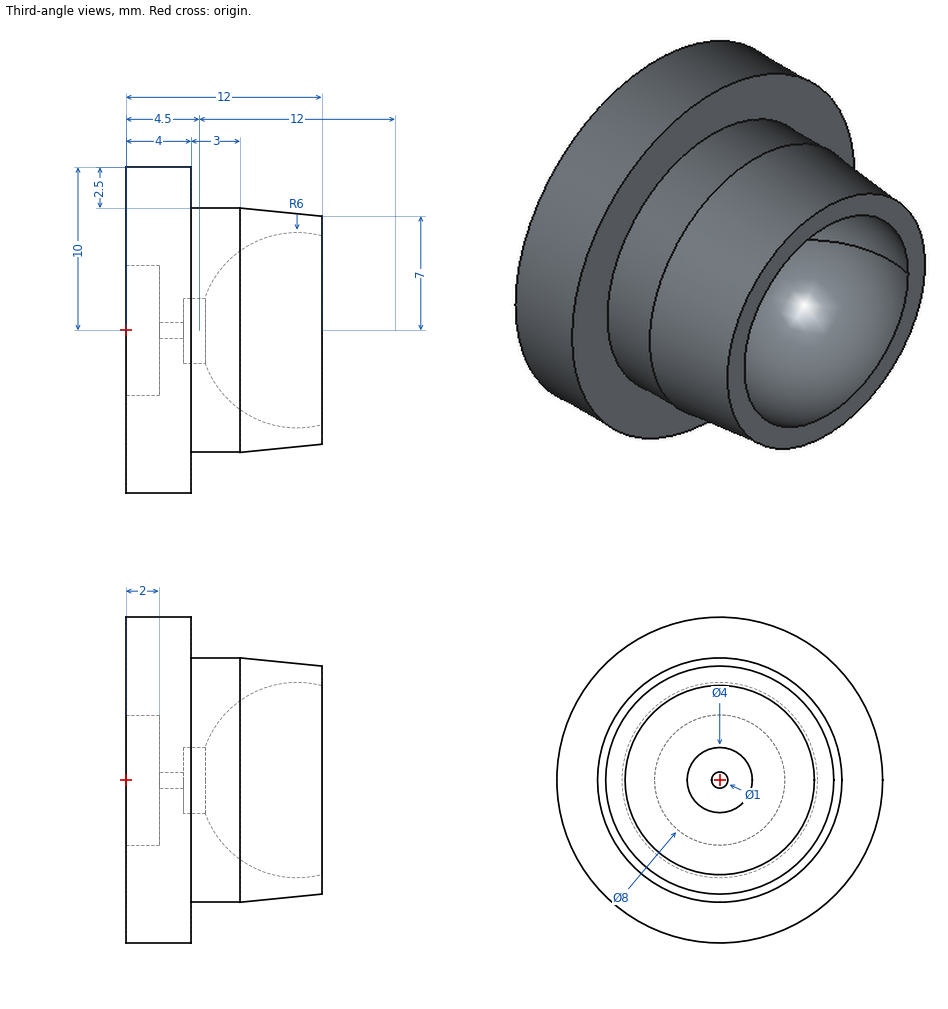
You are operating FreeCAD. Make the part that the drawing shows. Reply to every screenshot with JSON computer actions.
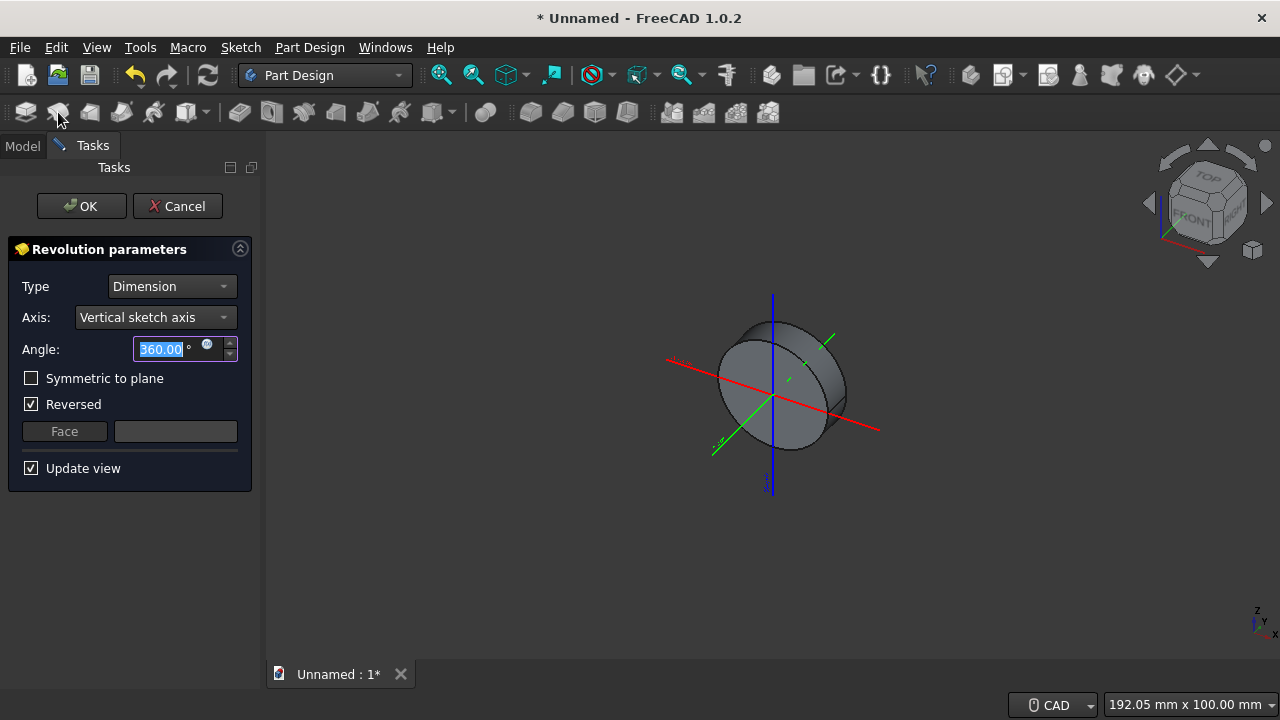
{"action": "left_click", "coordinate": [156, 318]}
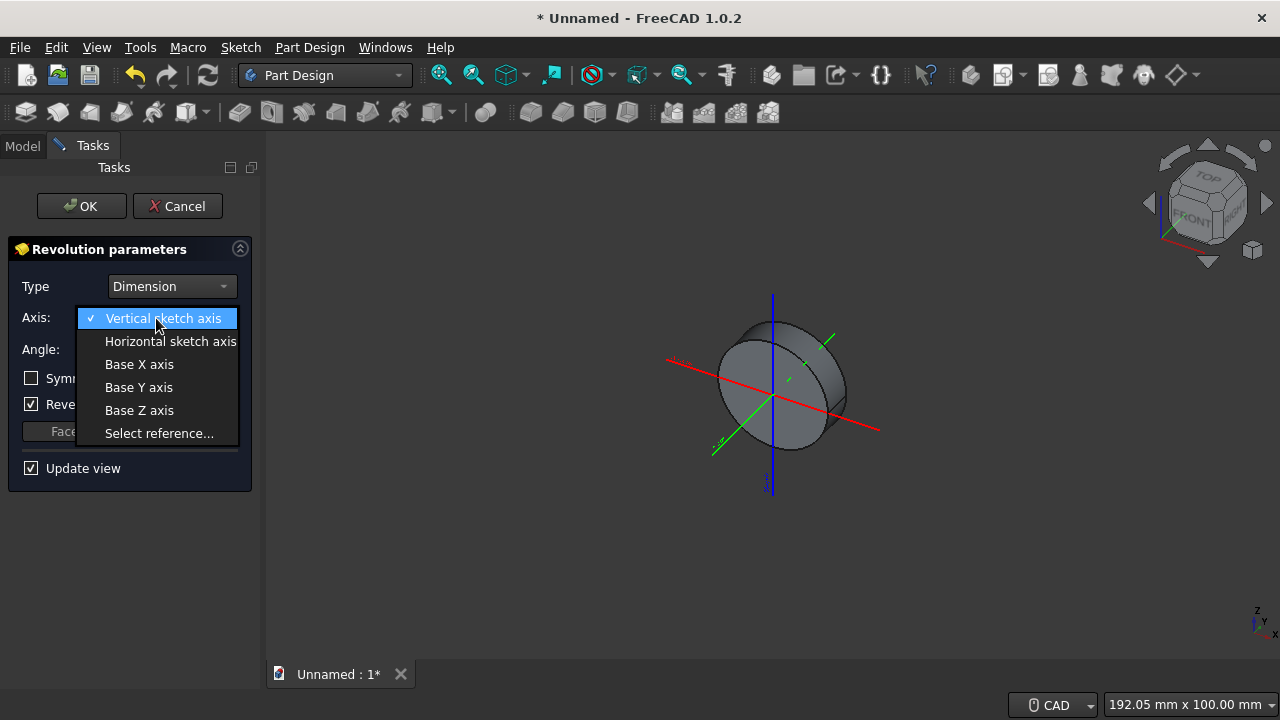
{"action": "left_click", "coordinate": [156, 342]}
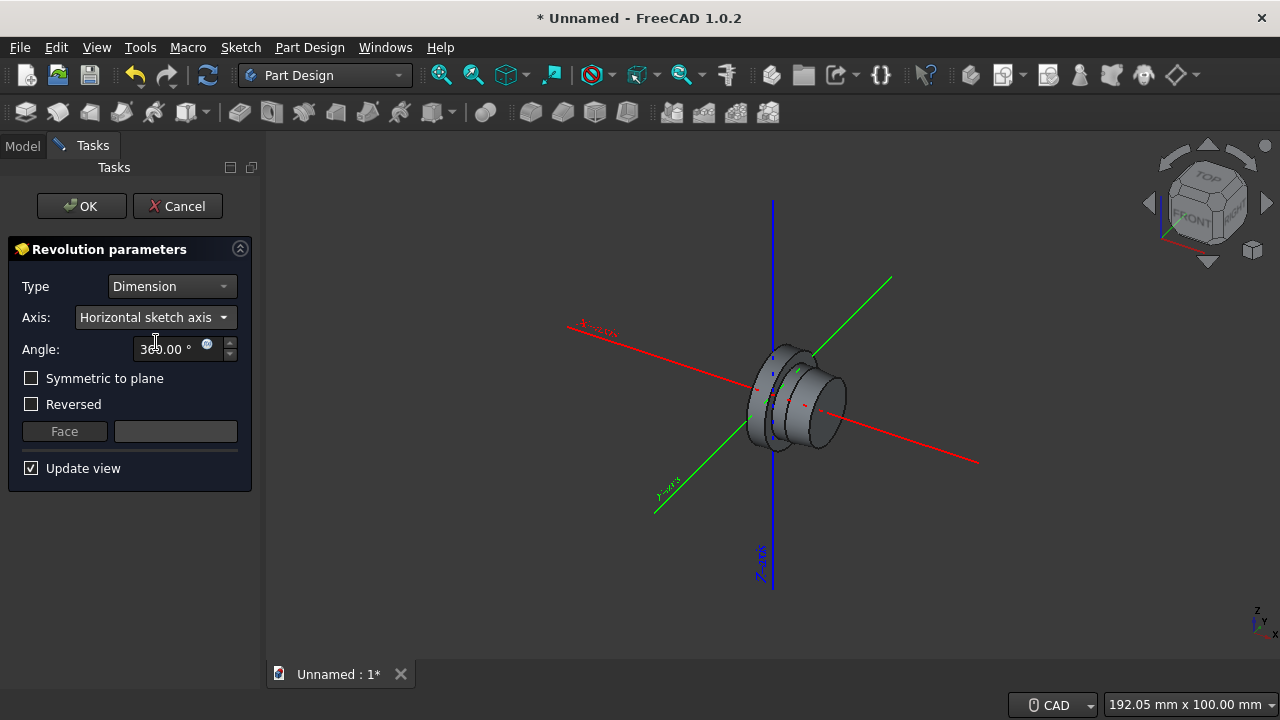
{"action": "left_click", "coordinate": [82, 206]}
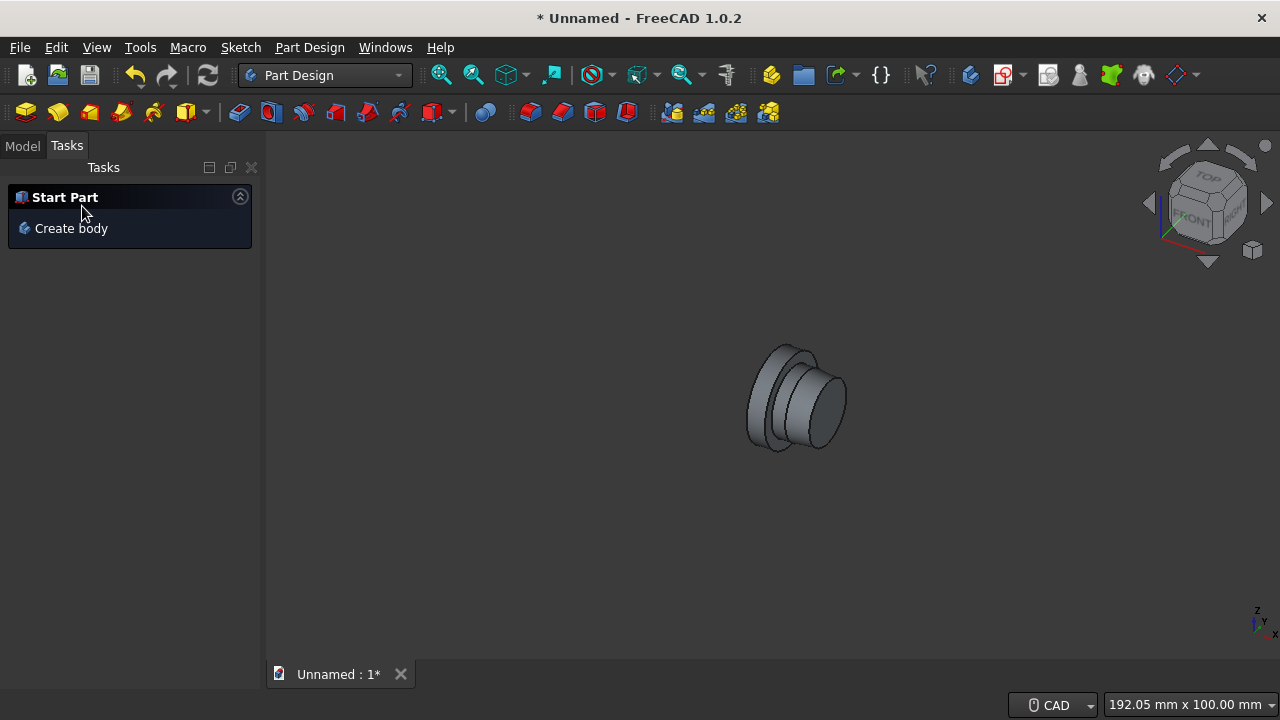
{"action": "left_click", "coordinate": [442, 76]}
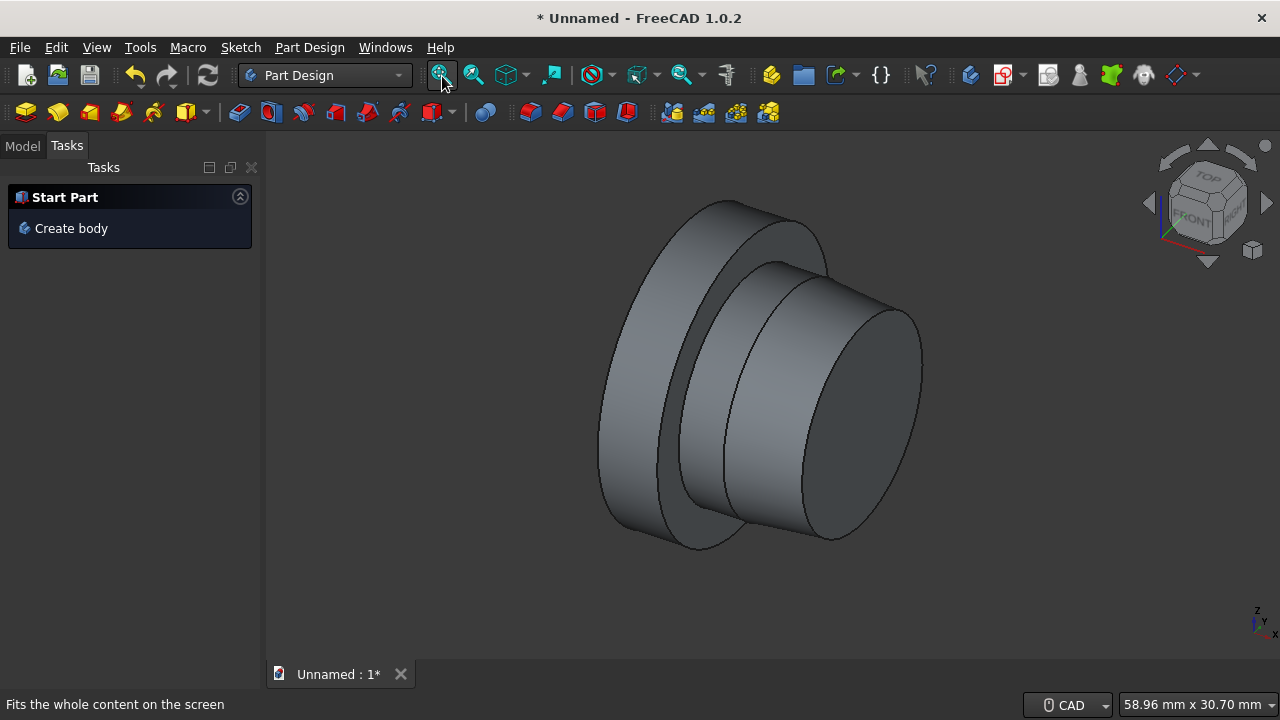
{"action": "key", "text": "6"}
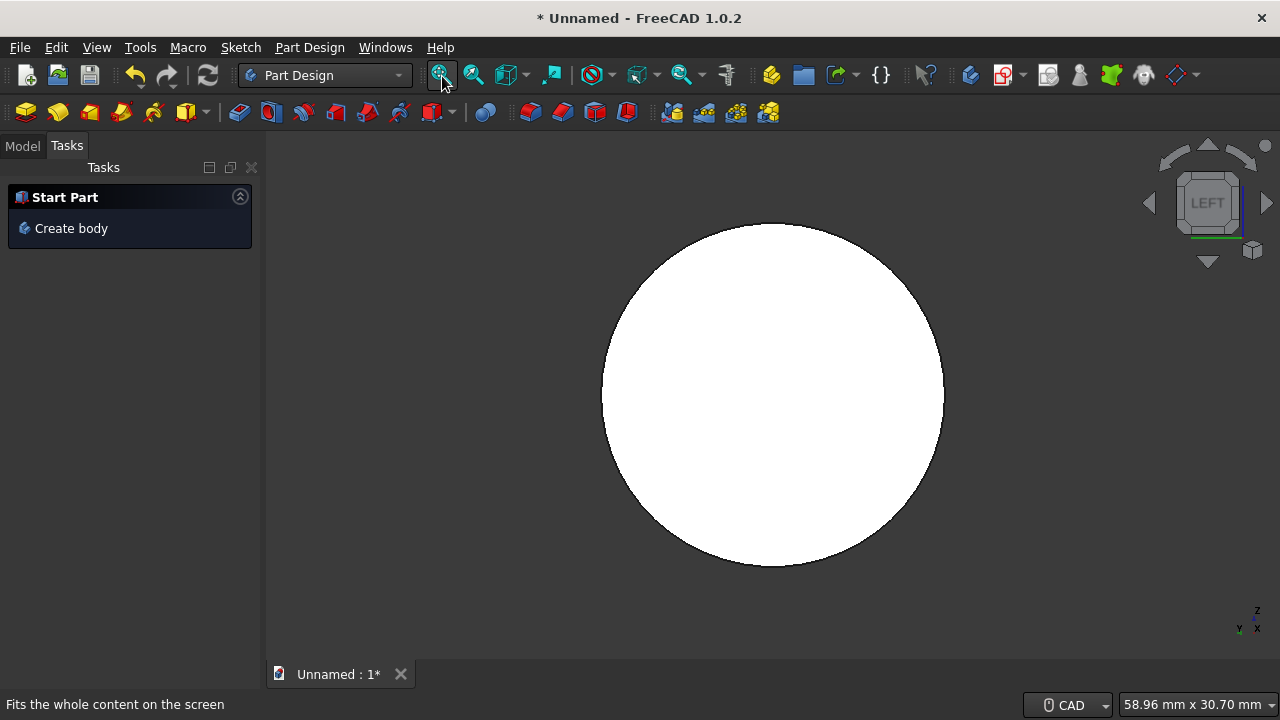
{"action": "left_click", "coordinate": [773, 394]}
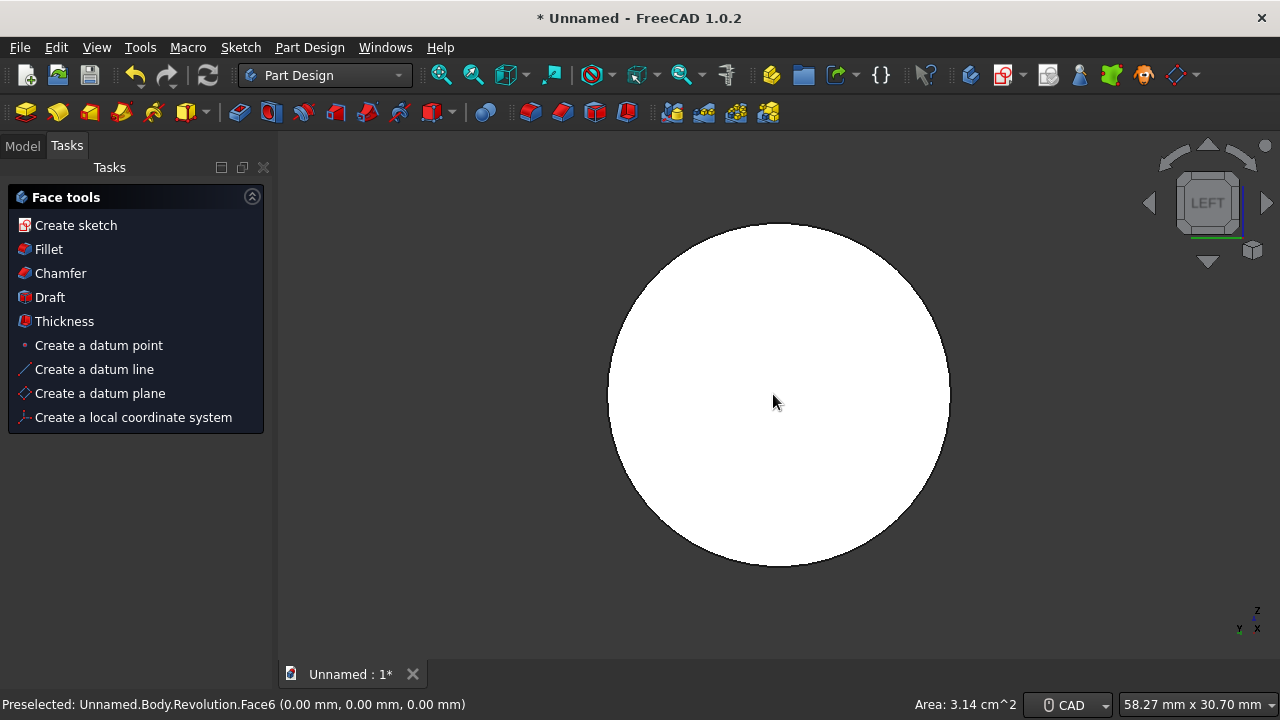
{"action": "left_click", "coordinate": [1004, 76]}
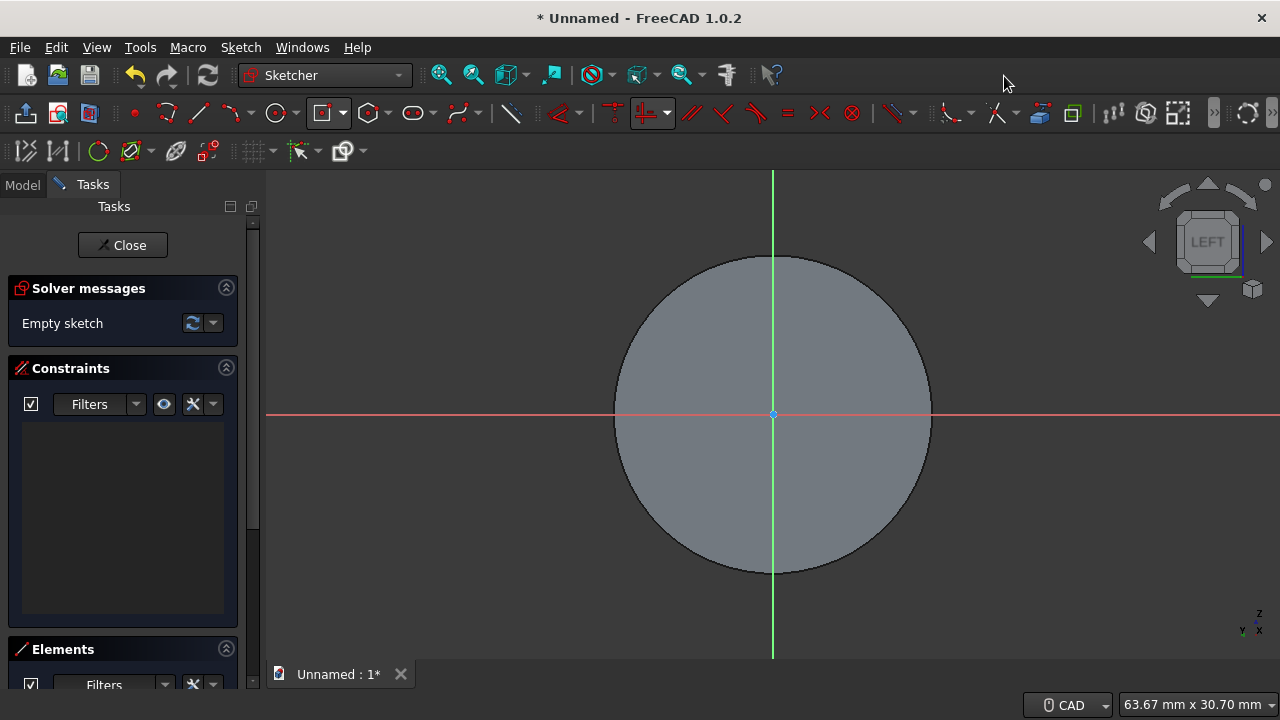
{"action": "scroll", "coordinate": [829, 414], "scroll_direction": "up", "scroll_amount": 4}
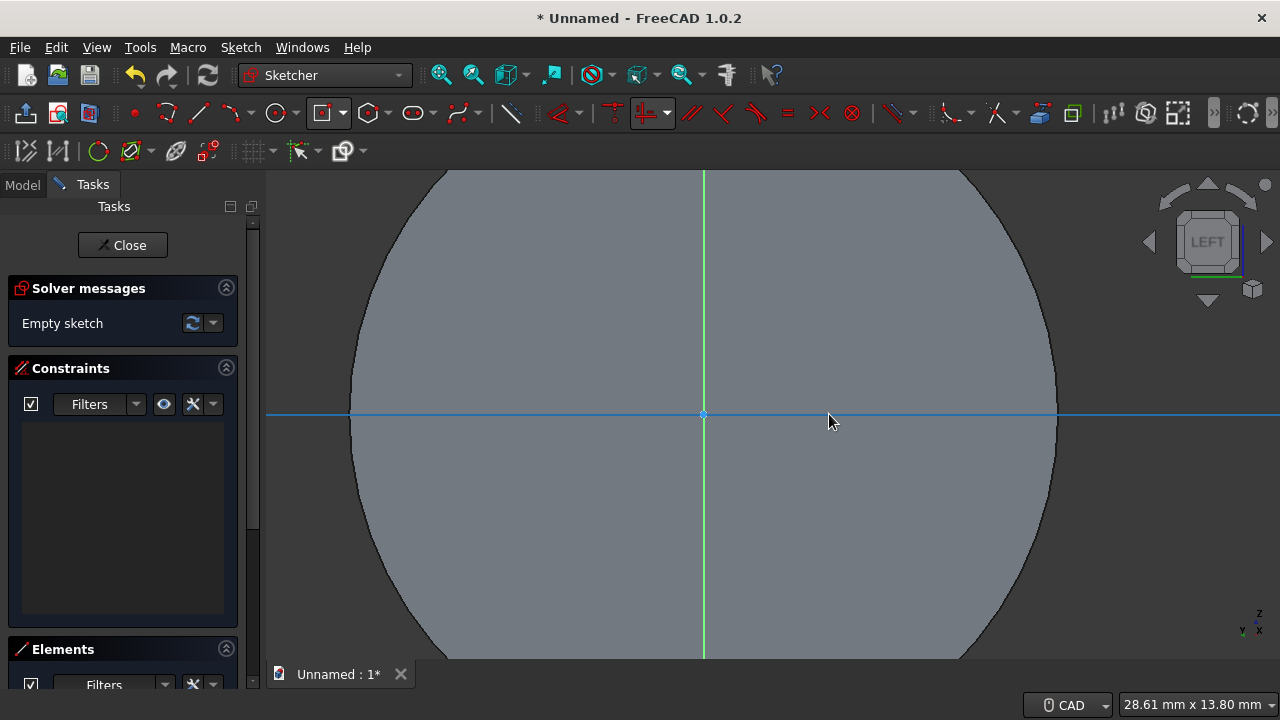
{"action": "left_click", "coordinate": [276, 114]}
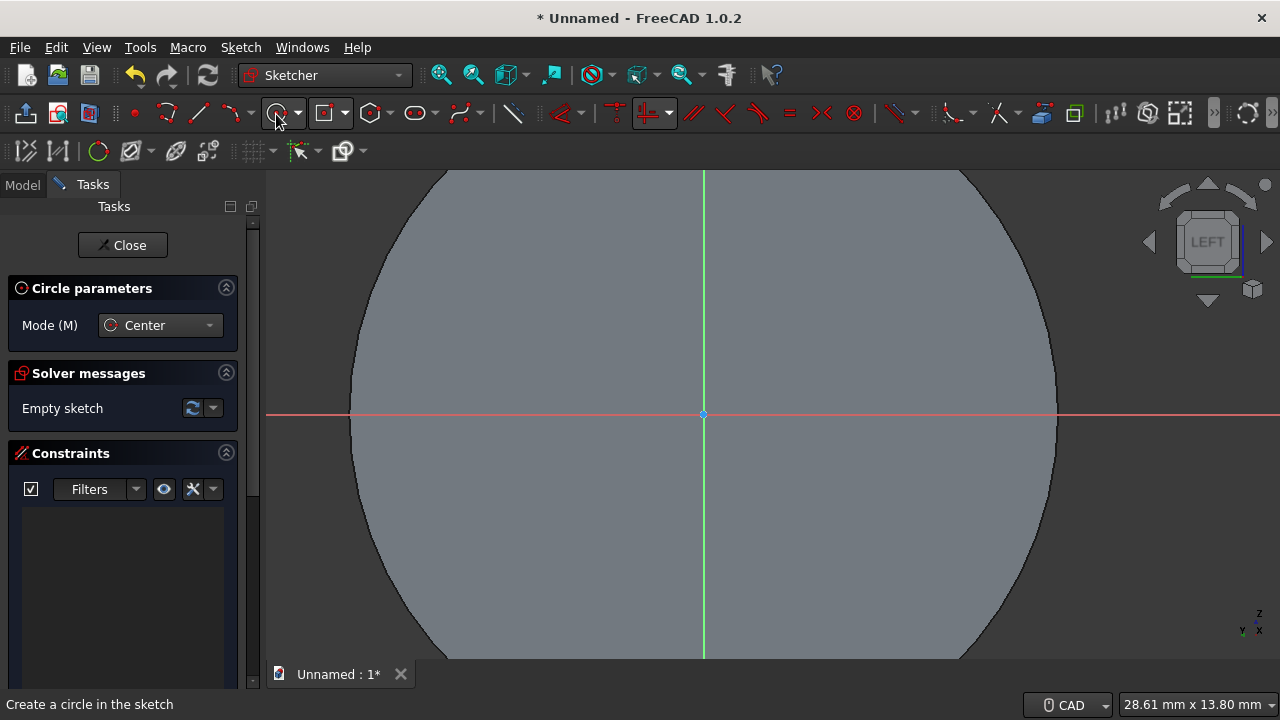
{"action": "left_click", "coordinate": [704, 414]}
{"action": "mouse_move", "coordinate": [804, 314]}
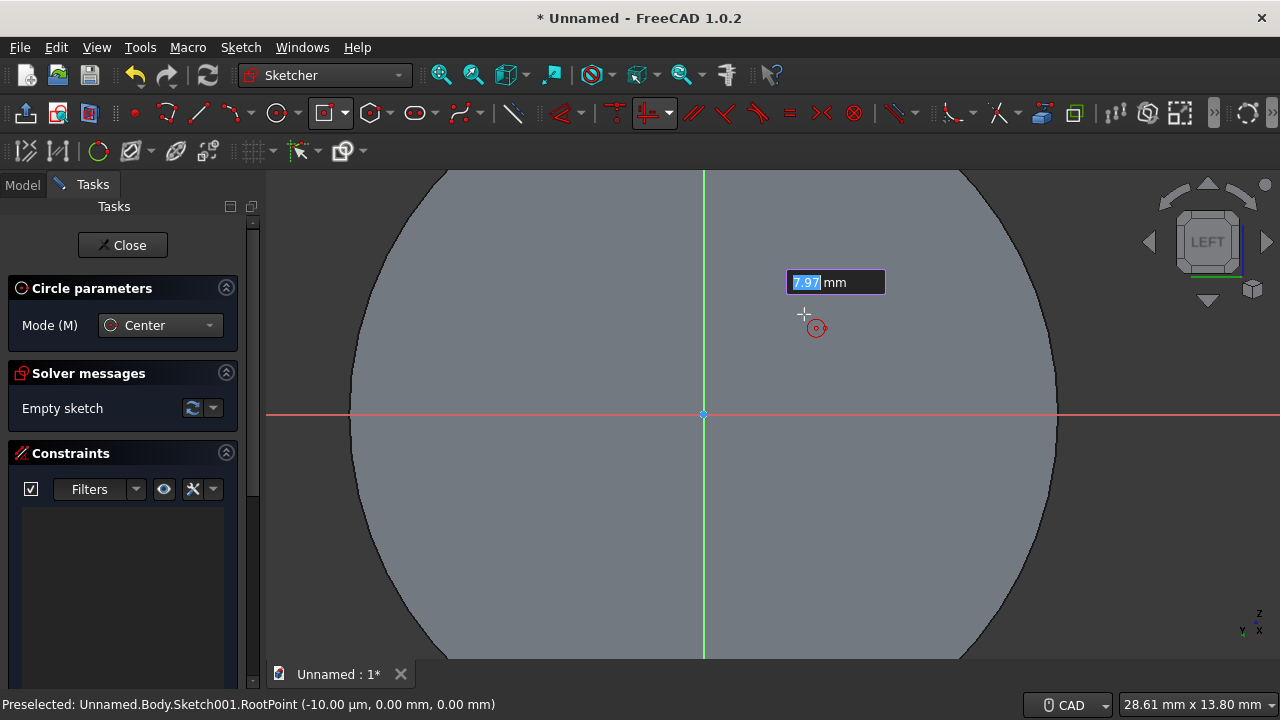
{"action": "type", "text": "8"}
{"action": "key", "text": "Return"}
{"action": "key", "text": "Escape"}